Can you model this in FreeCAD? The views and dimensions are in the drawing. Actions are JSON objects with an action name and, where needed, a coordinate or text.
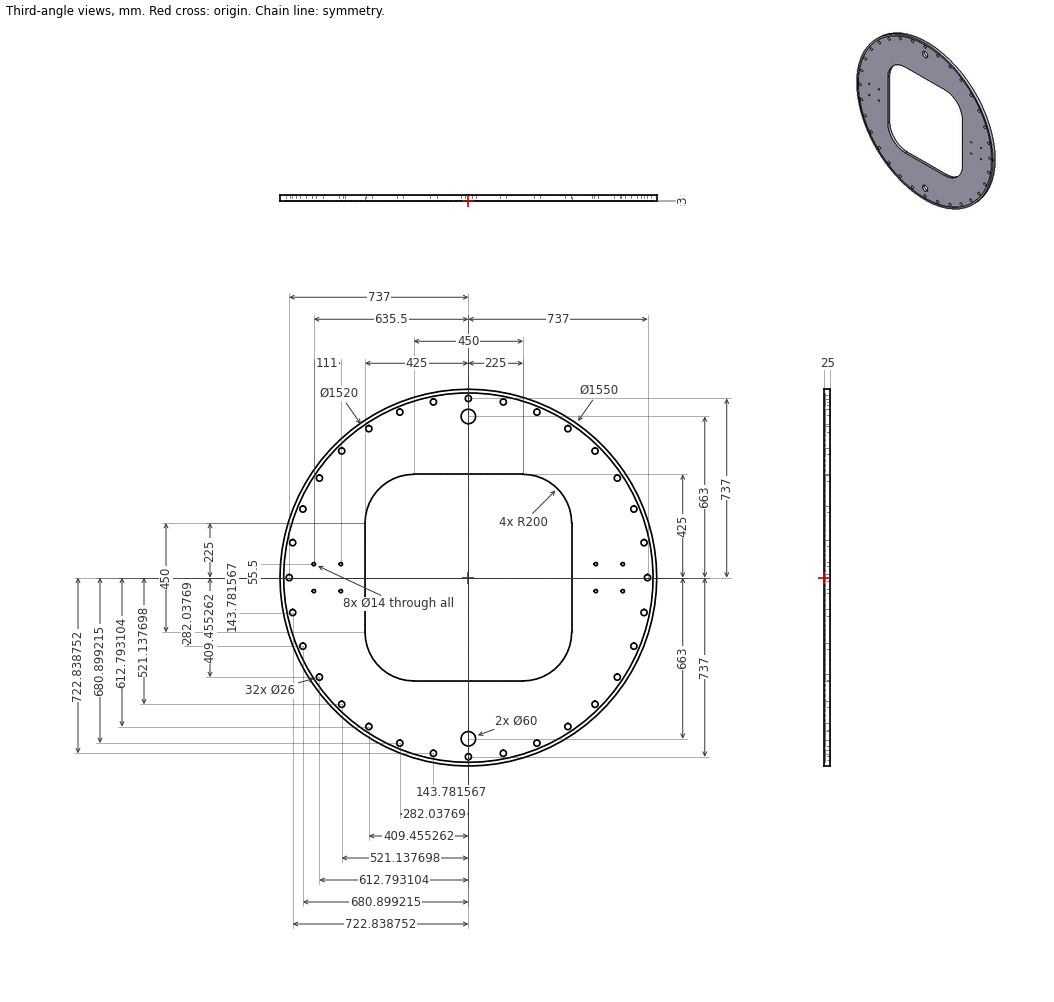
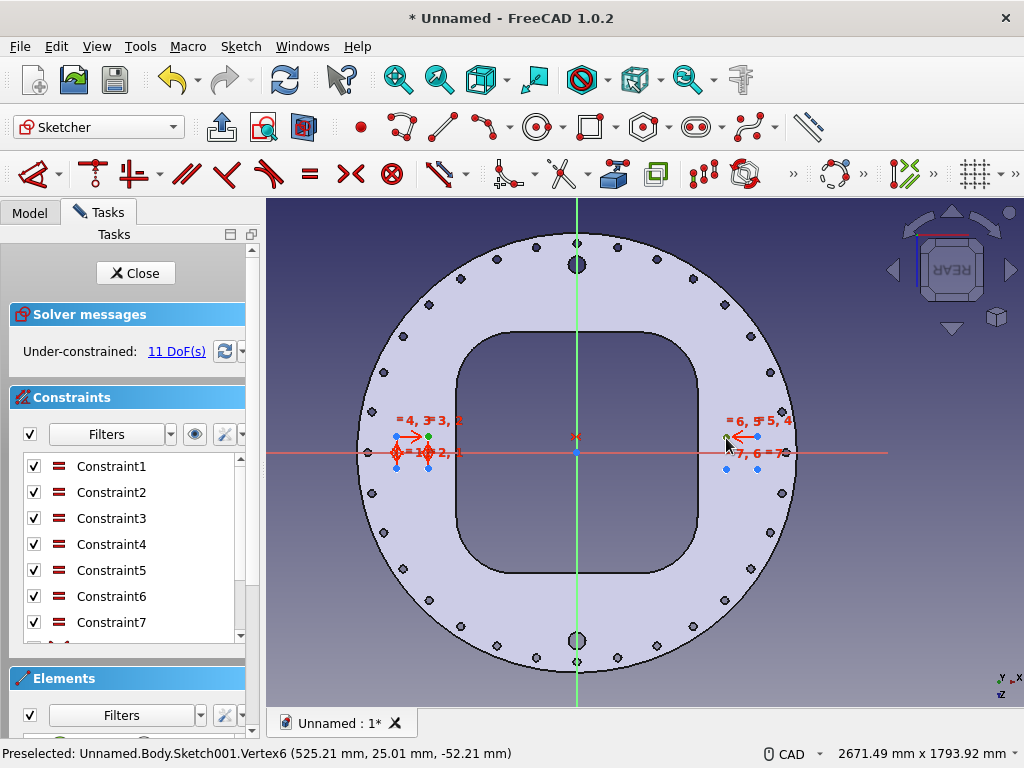
{"action": "left_click", "coordinate": [577, 647]}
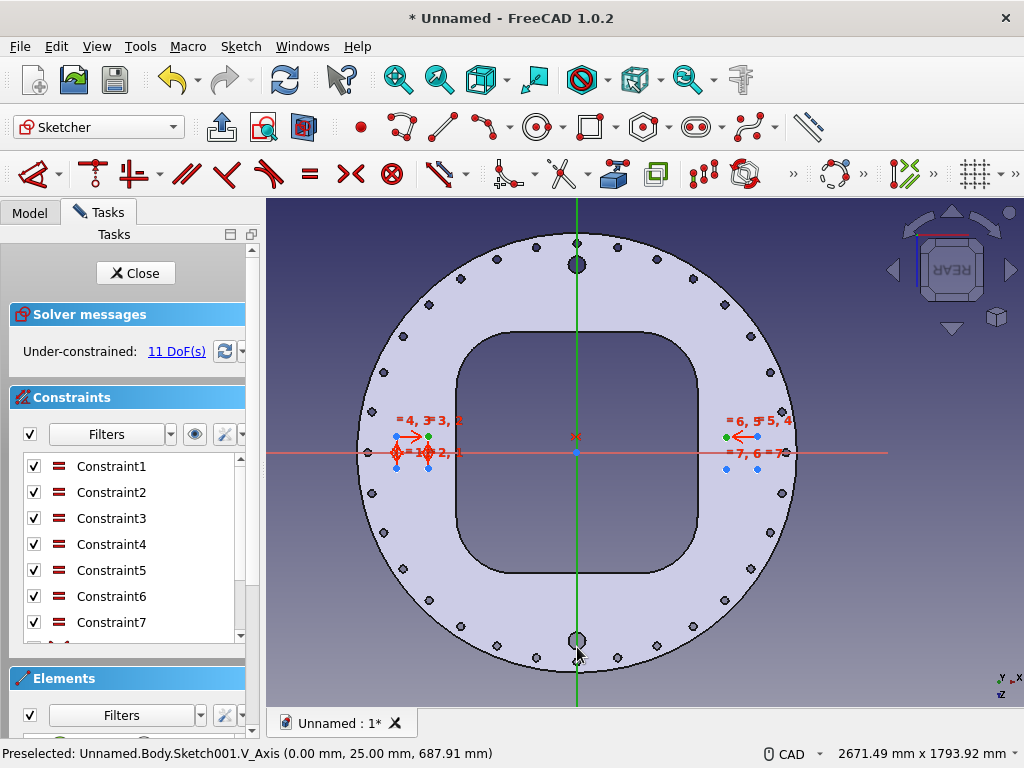
{"action": "left_click", "coordinate": [351, 174]}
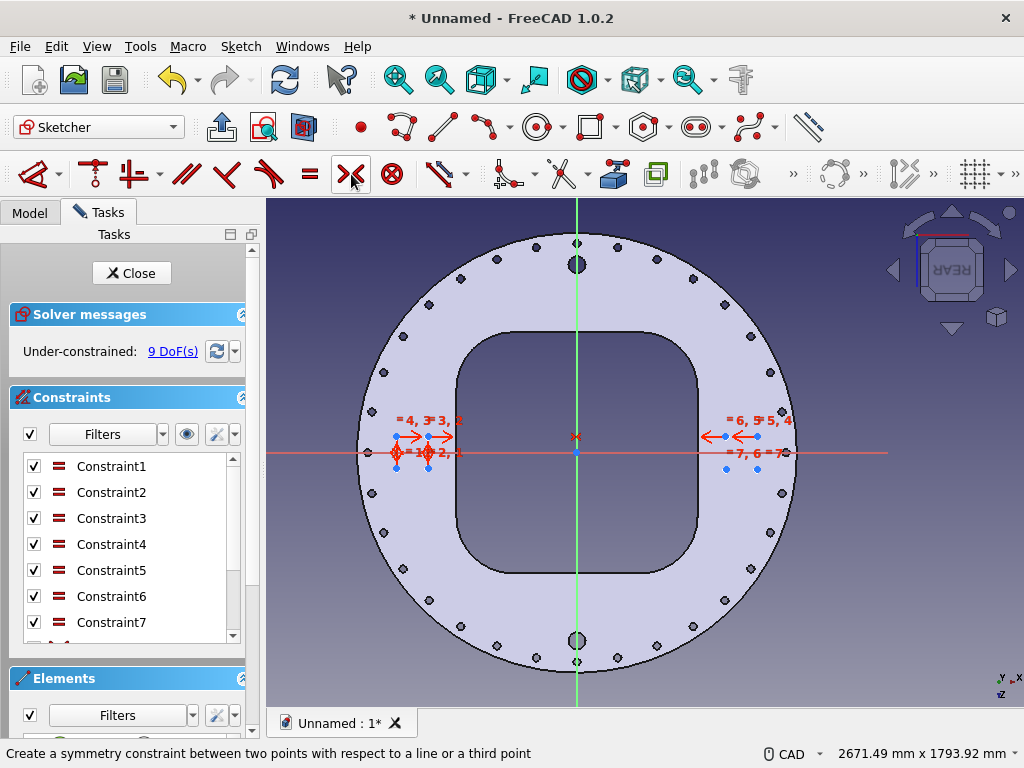
{"action": "left_click", "coordinate": [428, 469]}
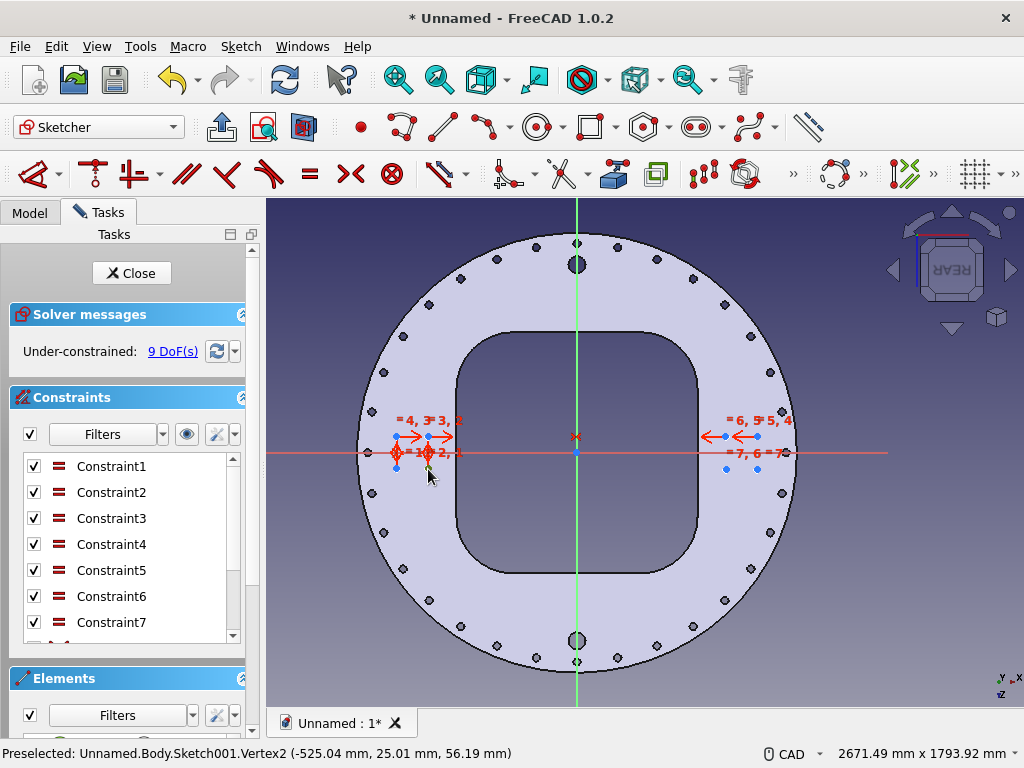
{"action": "left_click", "coordinate": [726, 470]}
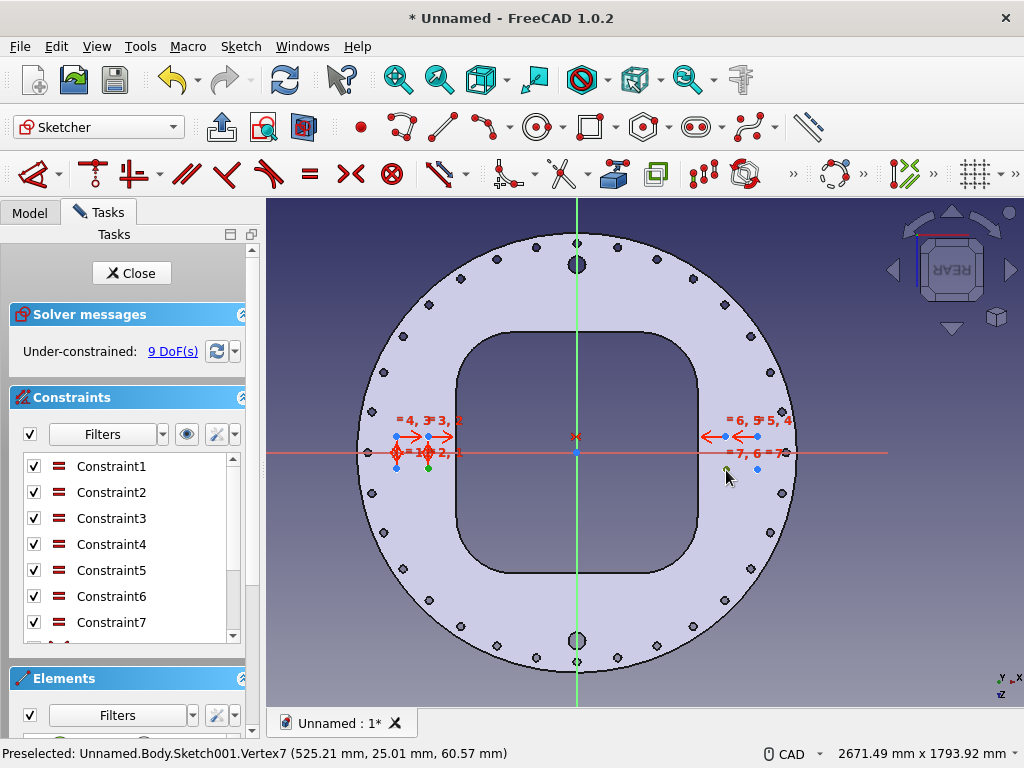
{"action": "left_click", "coordinate": [577, 647]}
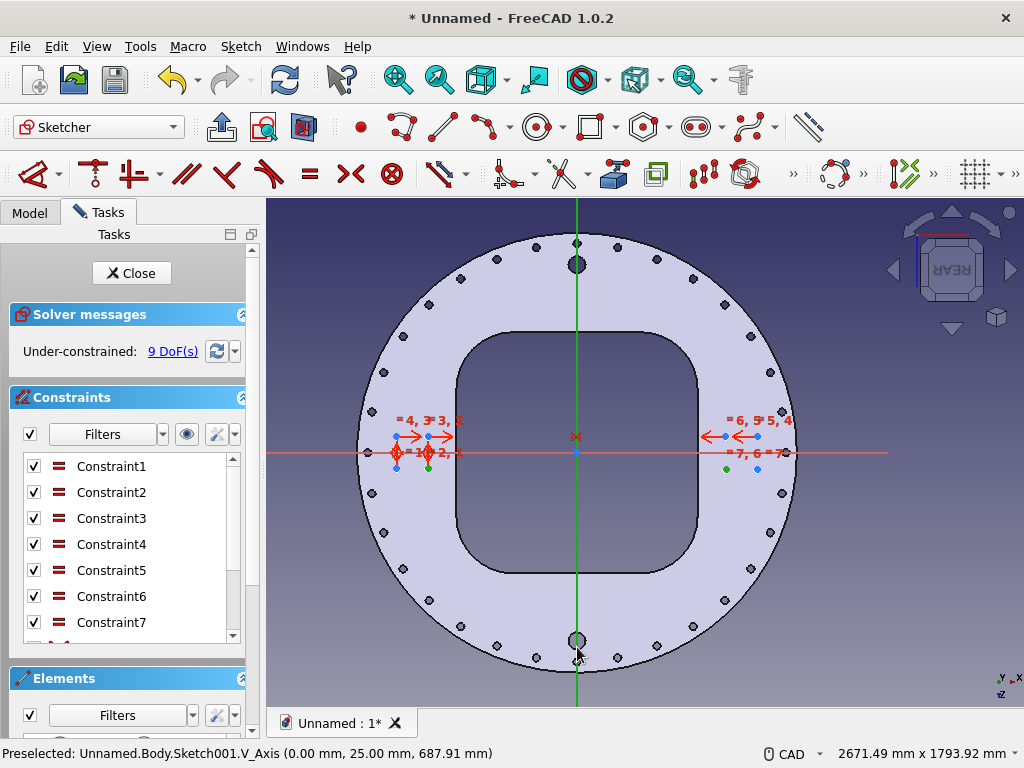
{"action": "left_click", "coordinate": [351, 174]}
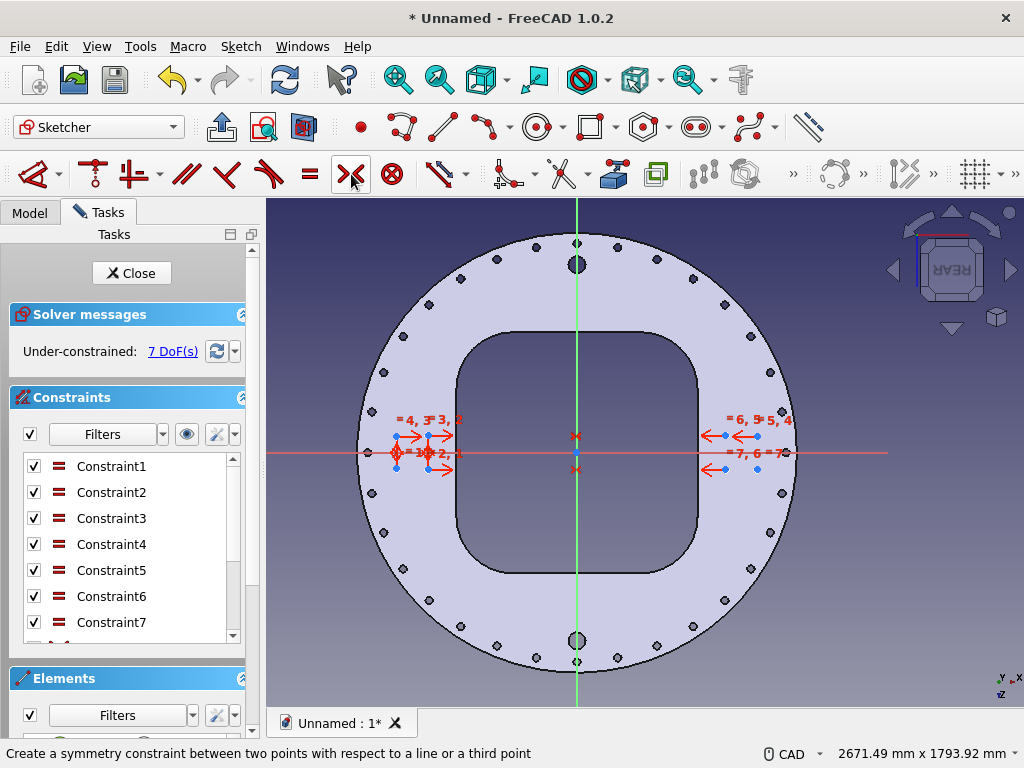
{"action": "left_click", "coordinate": [397, 469]}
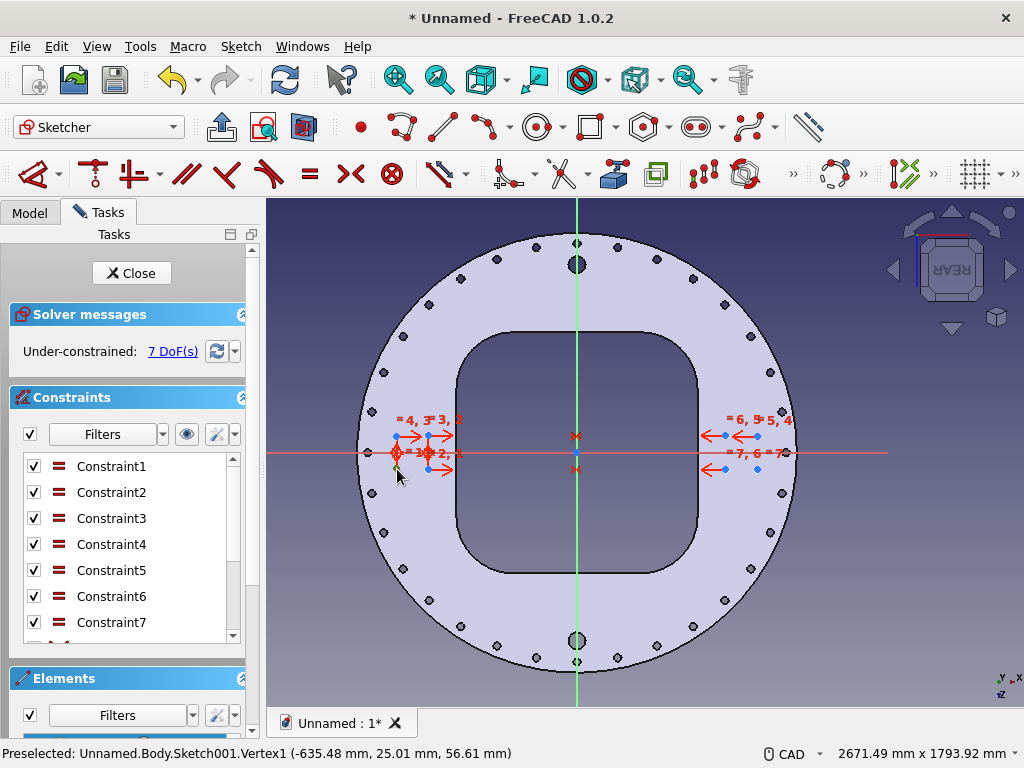
{"action": "left_click", "coordinate": [757, 470]}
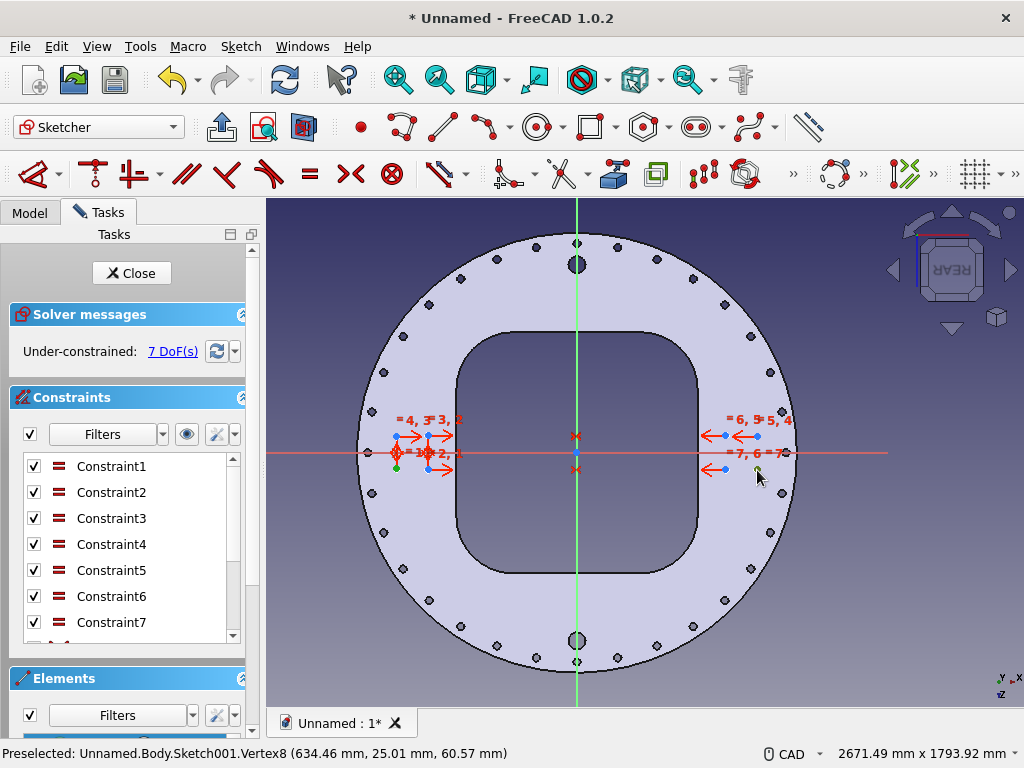
{"action": "left_click", "coordinate": [577, 647]}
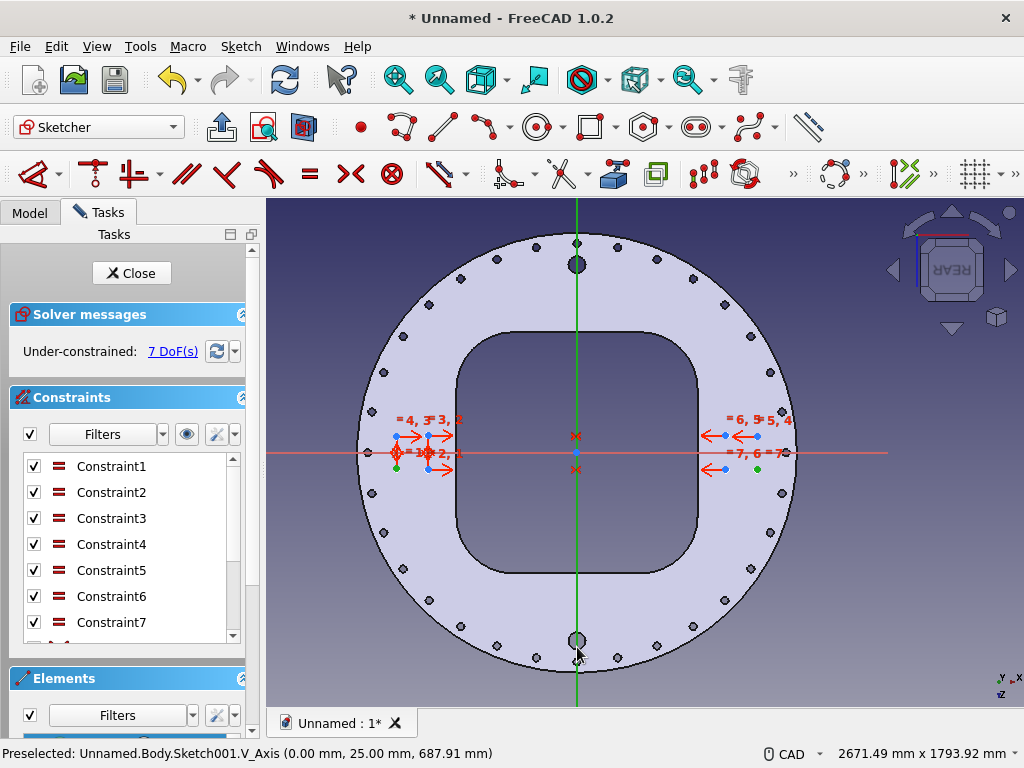
{"action": "left_click", "coordinate": [351, 174]}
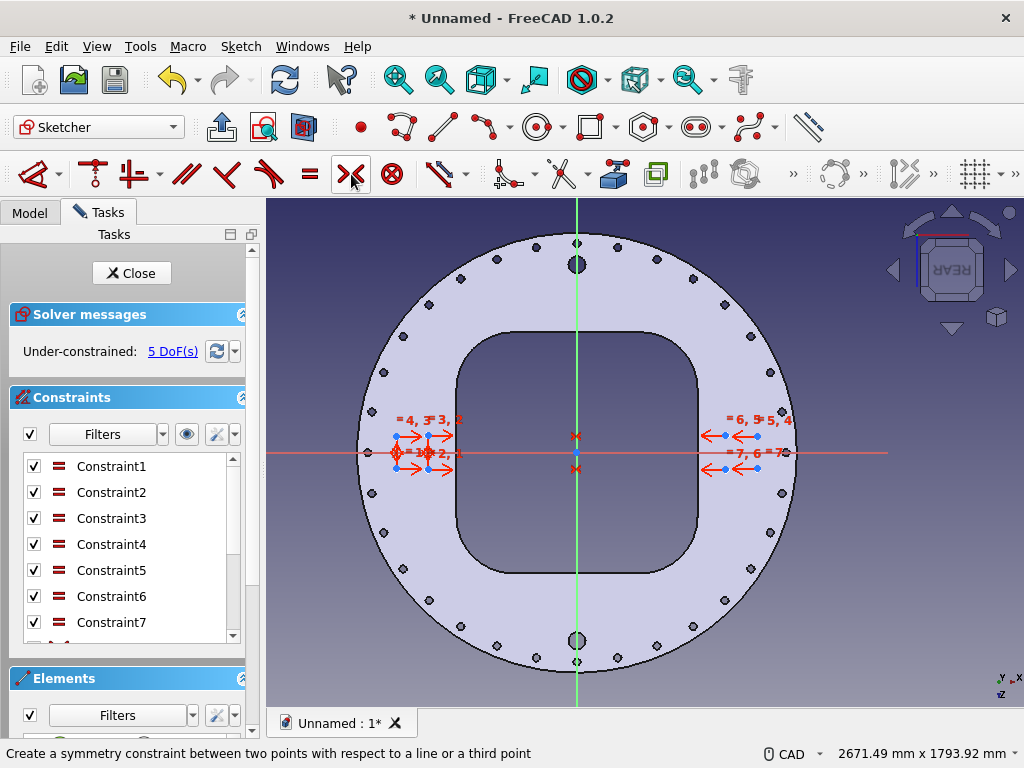
{"action": "left_click", "coordinate": [32, 174]}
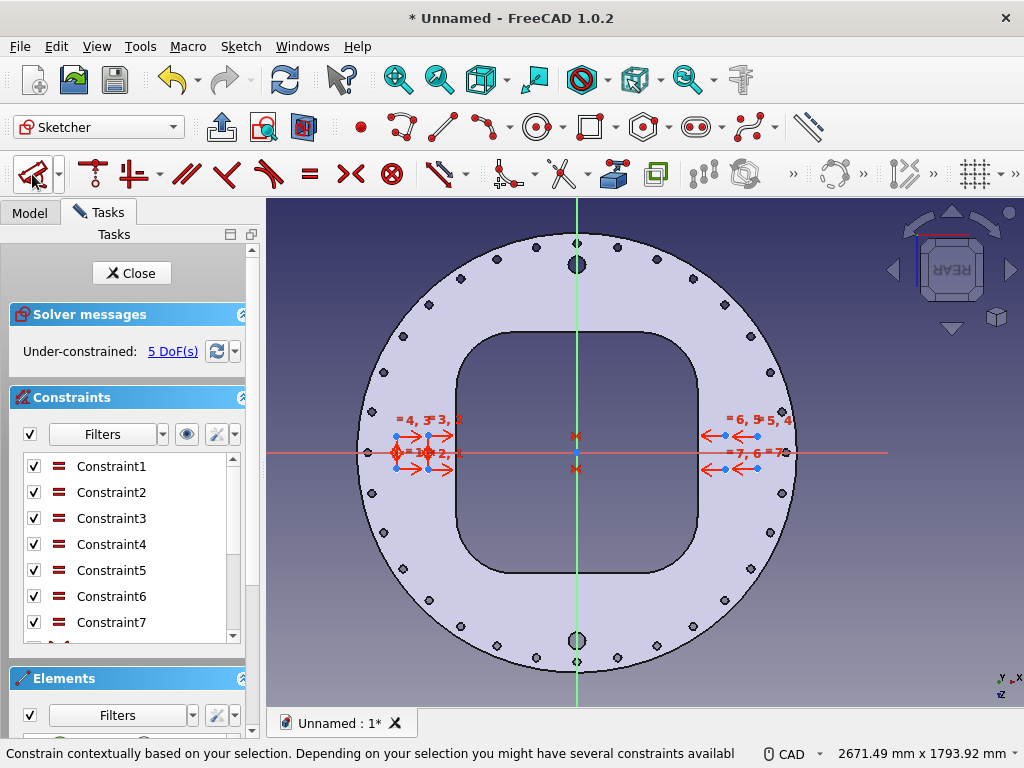
{"action": "scroll", "coordinate": [397, 466], "scroll_direction": "up", "scroll_amount": 12}